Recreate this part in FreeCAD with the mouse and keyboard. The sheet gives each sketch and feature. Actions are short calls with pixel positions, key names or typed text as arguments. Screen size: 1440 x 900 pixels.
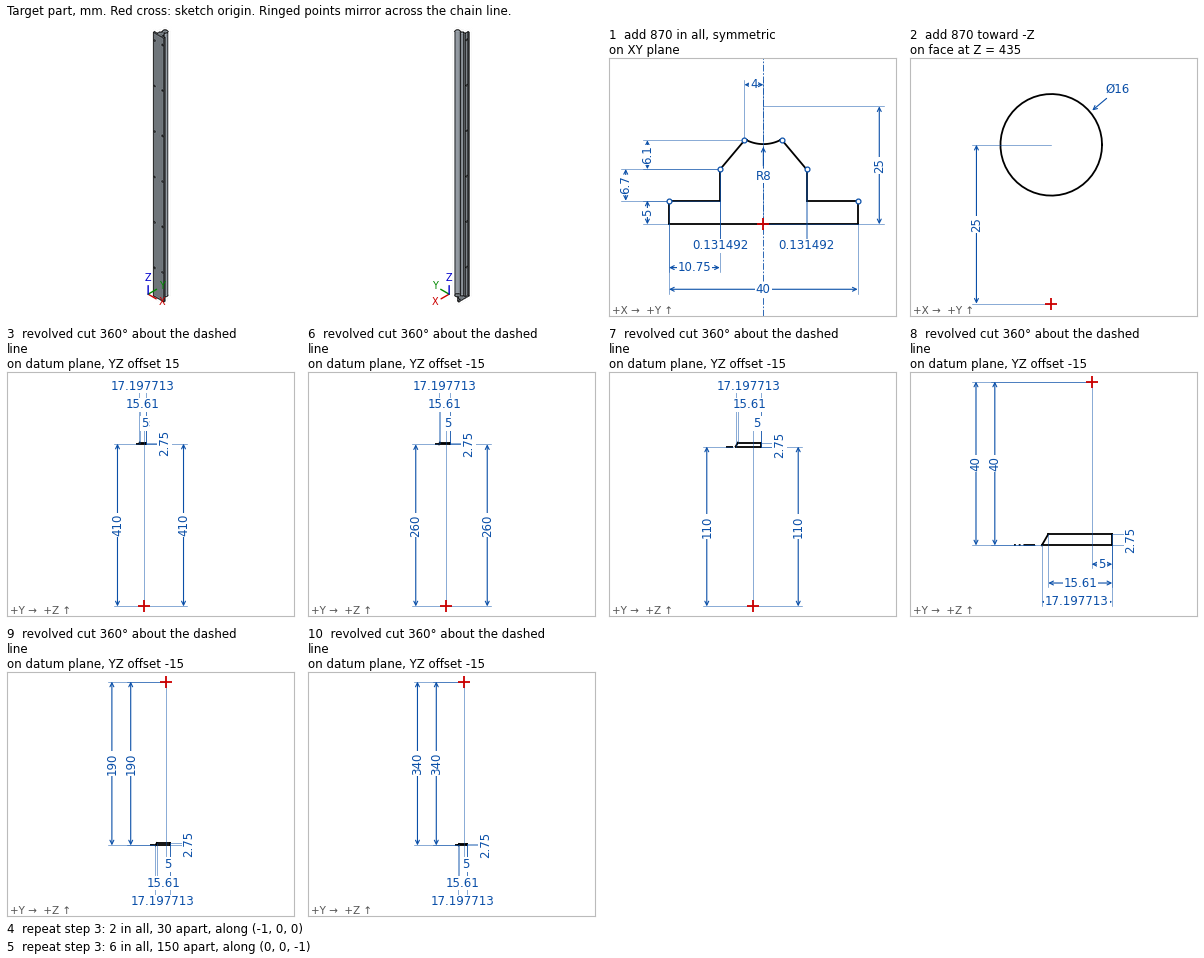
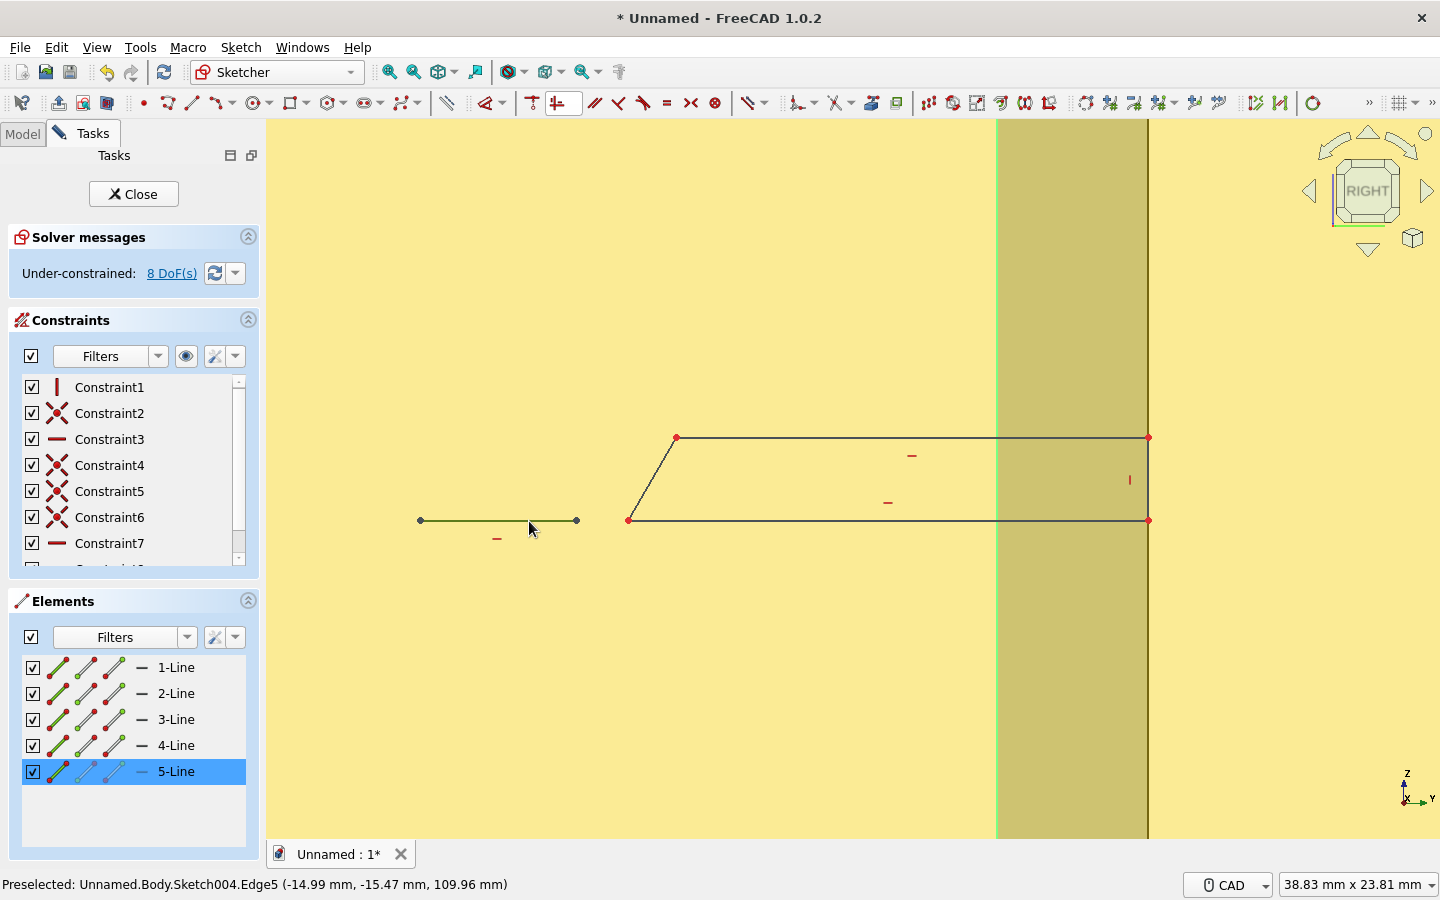
click(448, 104)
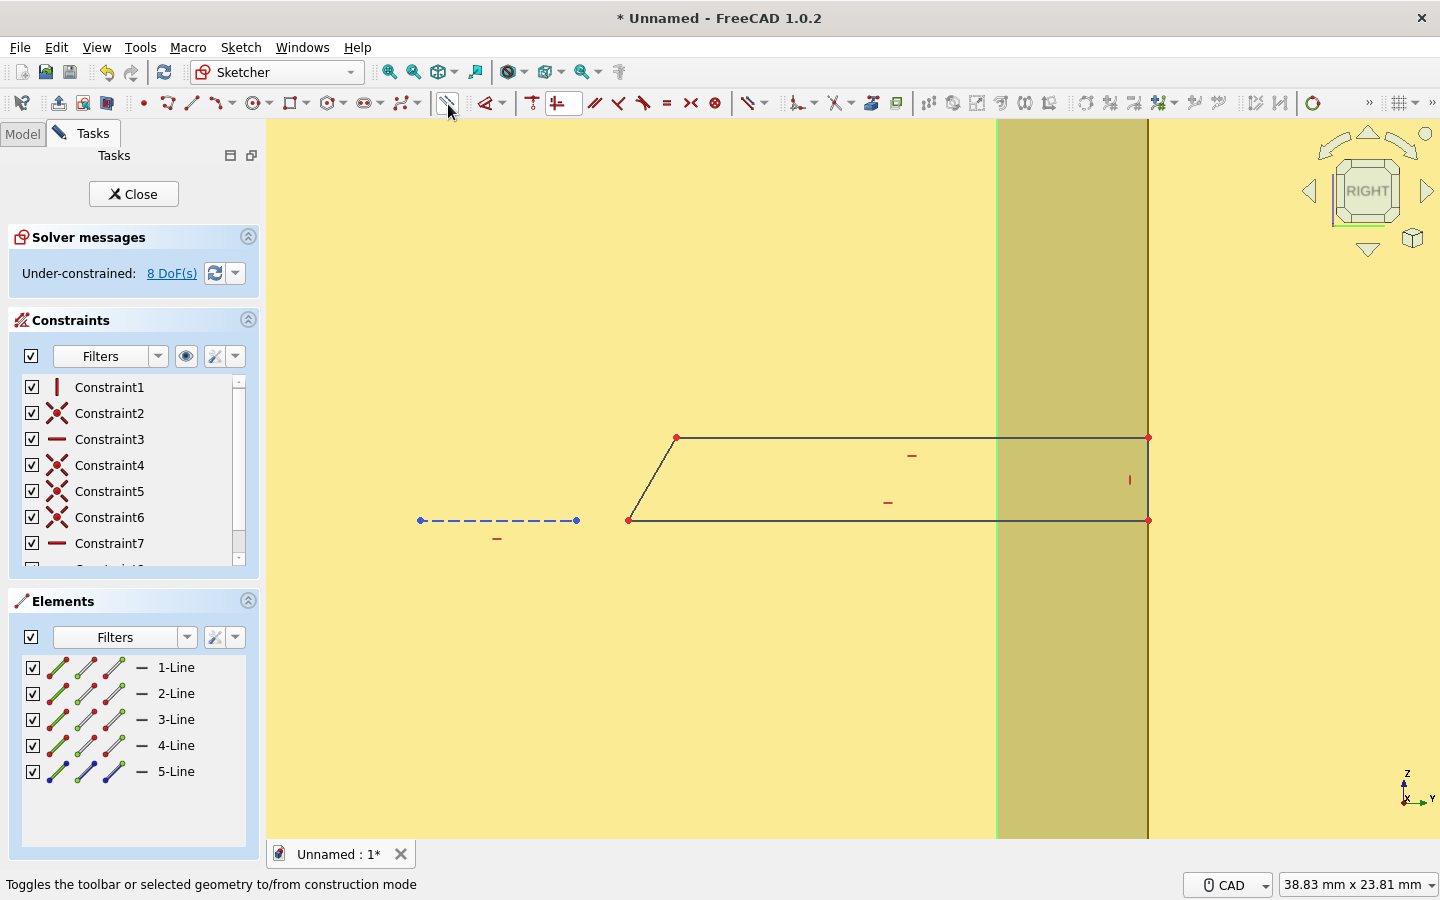
key(d)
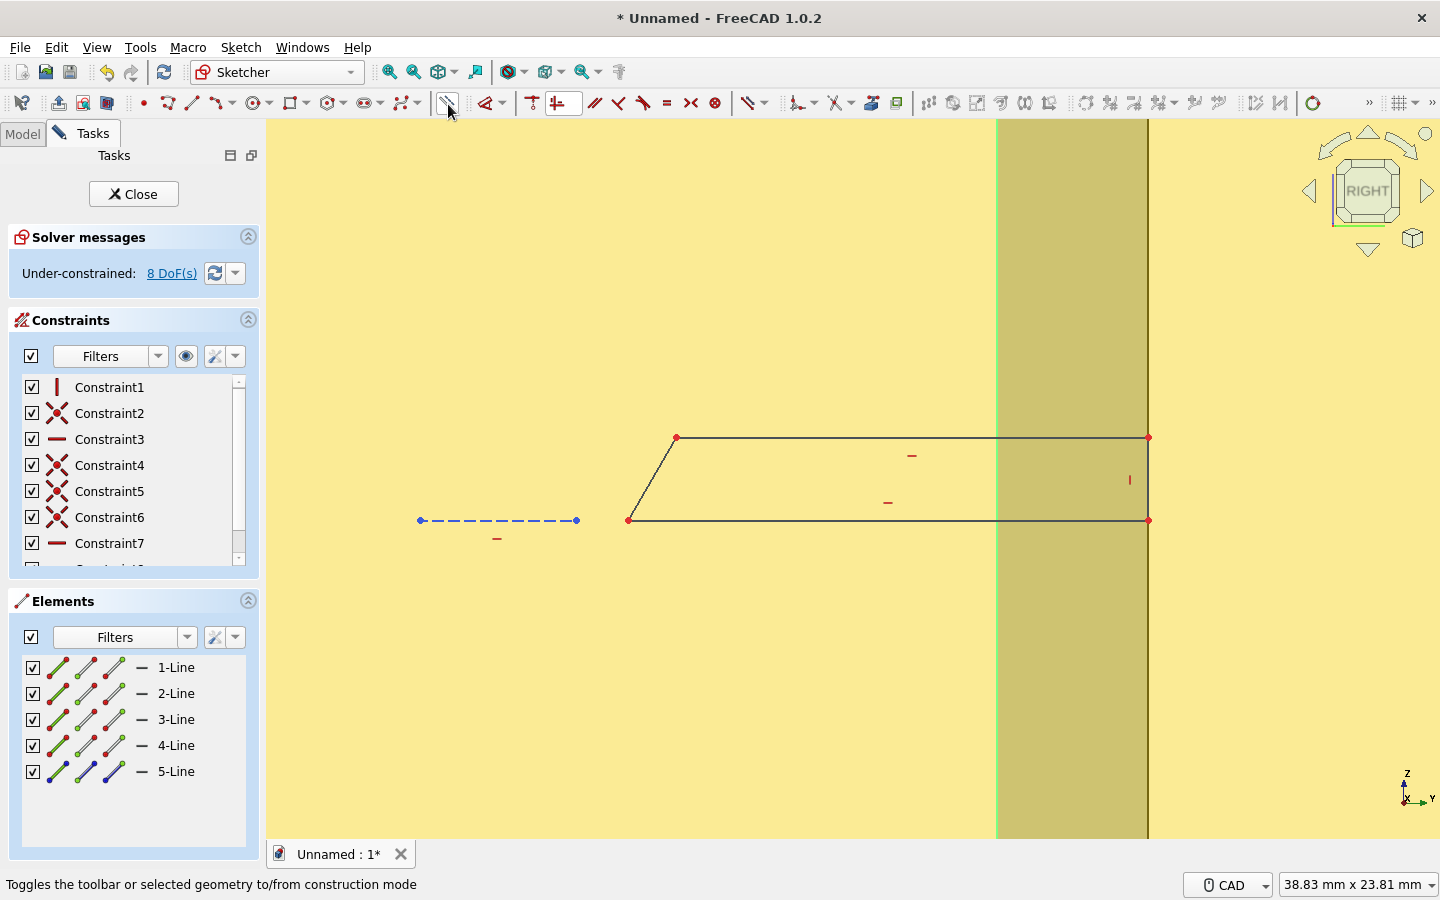
click(1148, 521)
click(1072, 487)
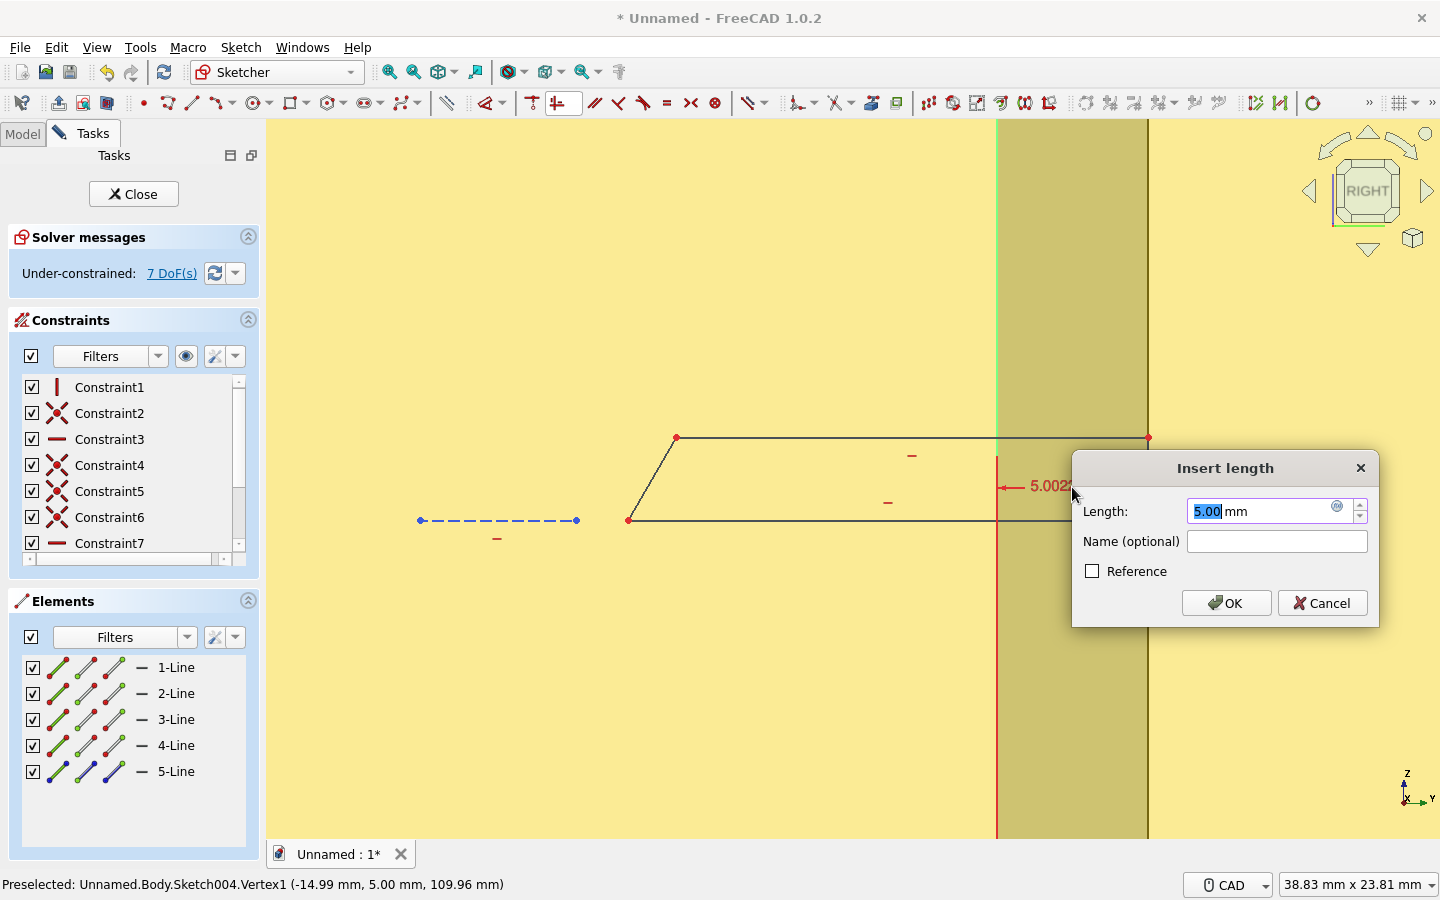
text(5)
key(Return)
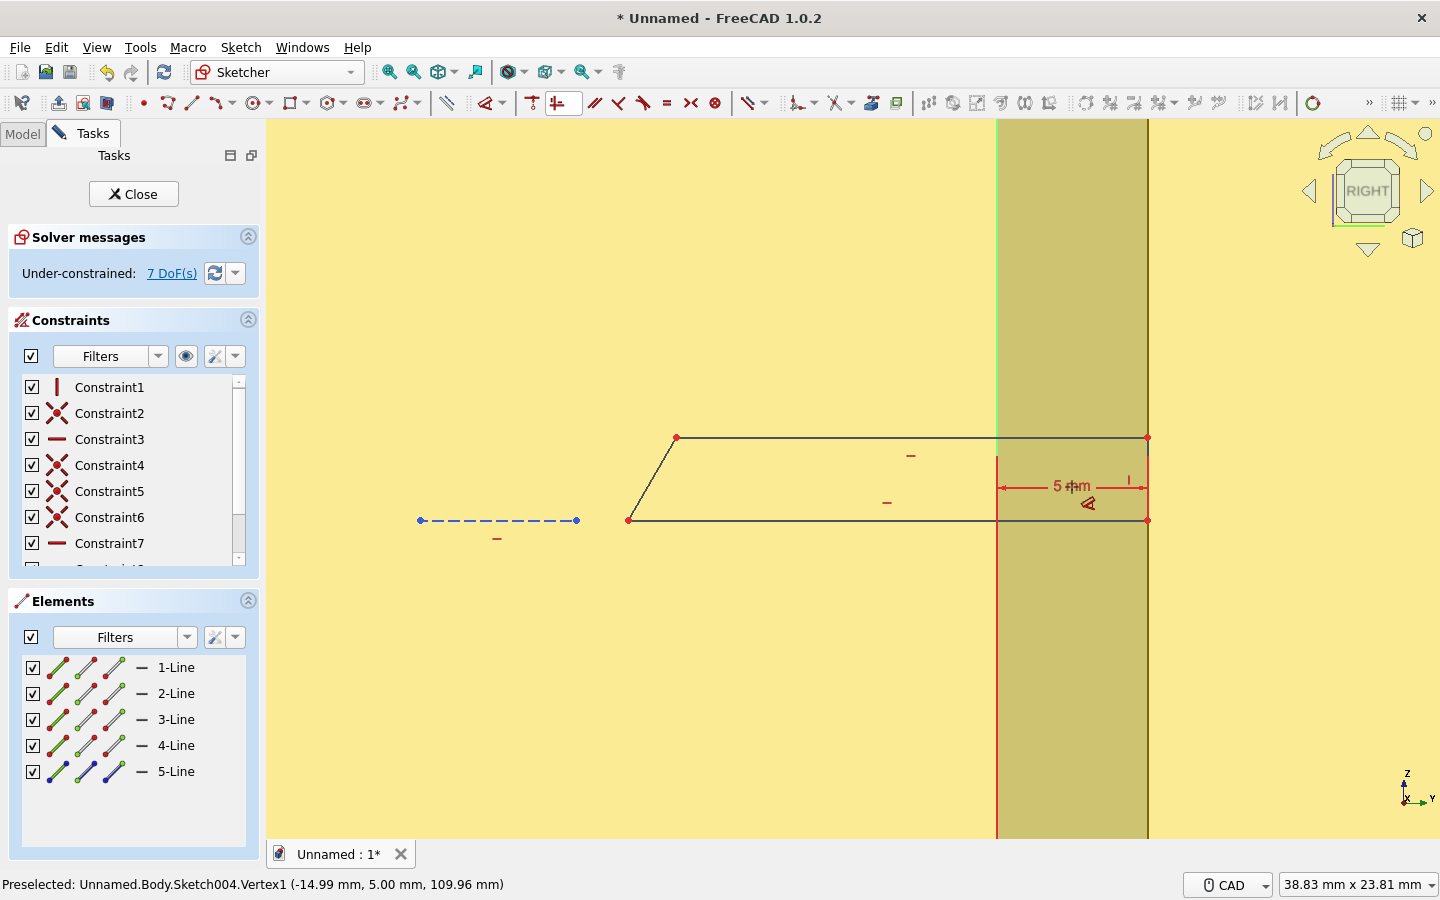
click(1148, 496)
click(1182, 479)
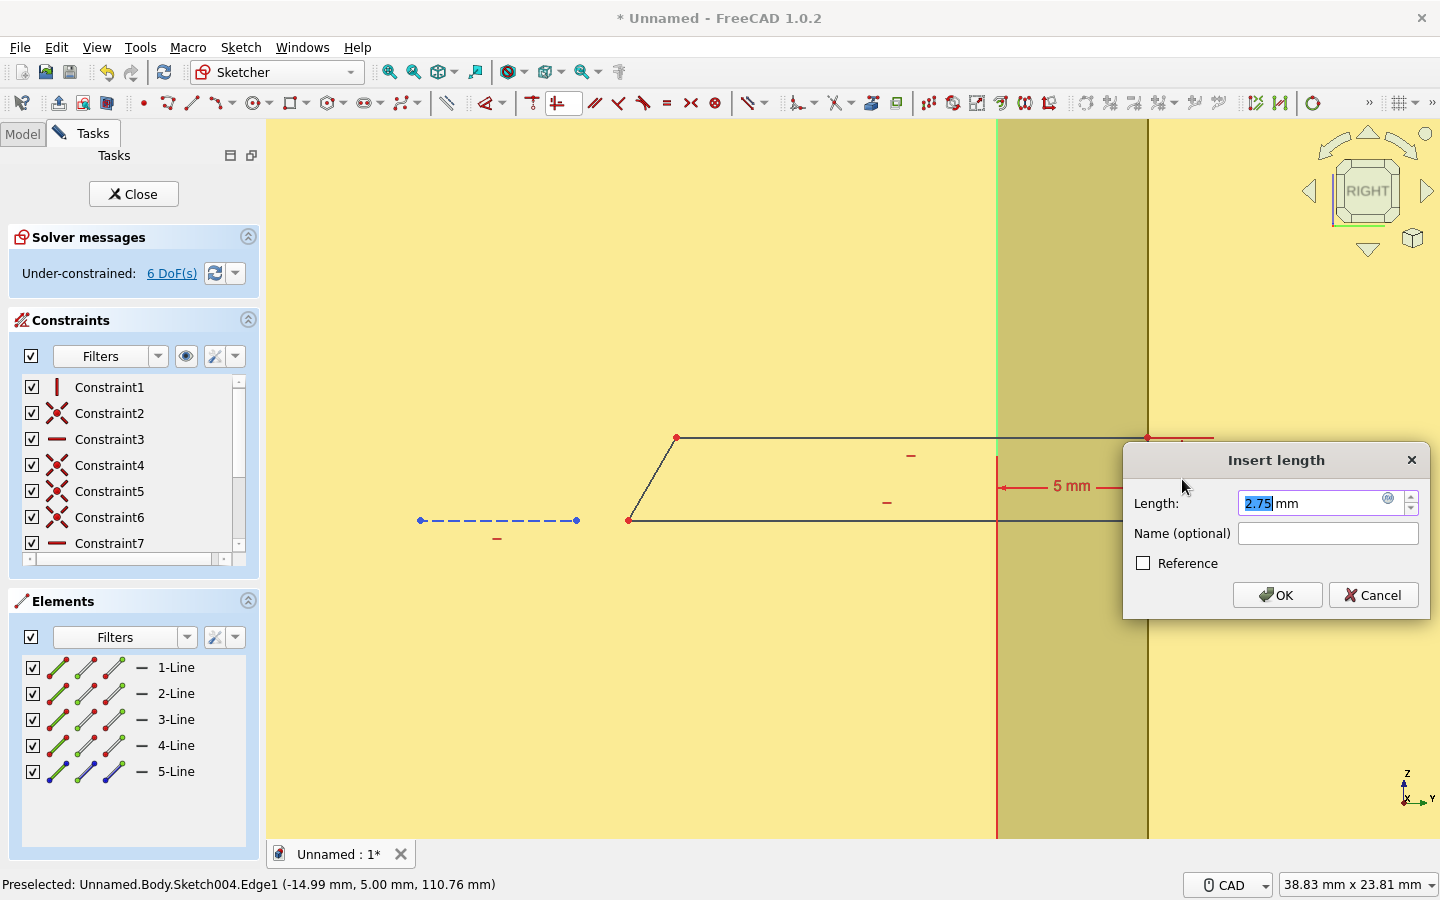
text(2.75)
key(Return)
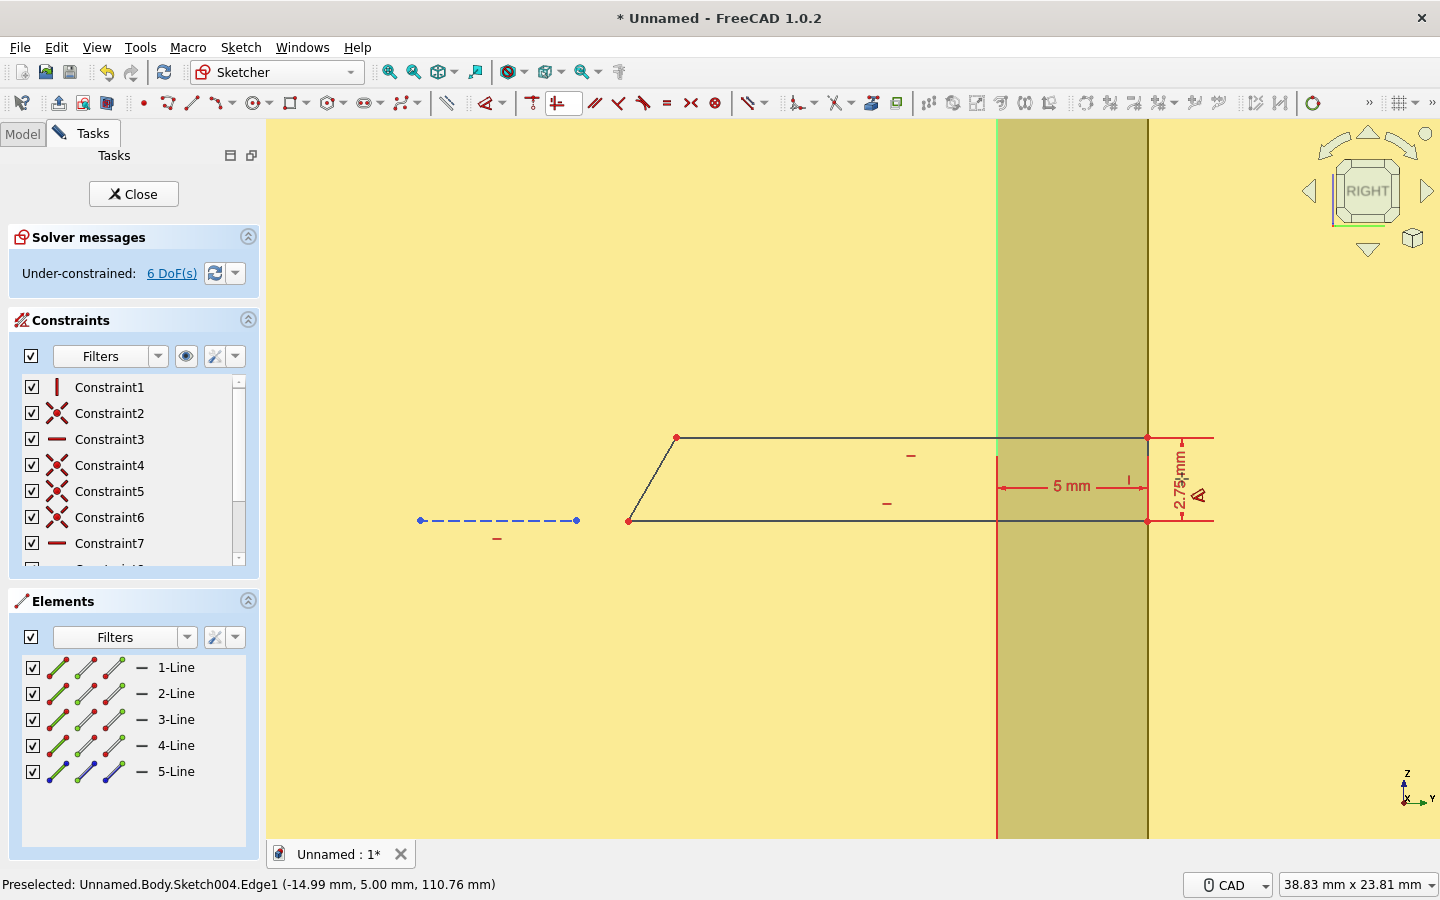
click(1148, 521)
click(1182, 666)